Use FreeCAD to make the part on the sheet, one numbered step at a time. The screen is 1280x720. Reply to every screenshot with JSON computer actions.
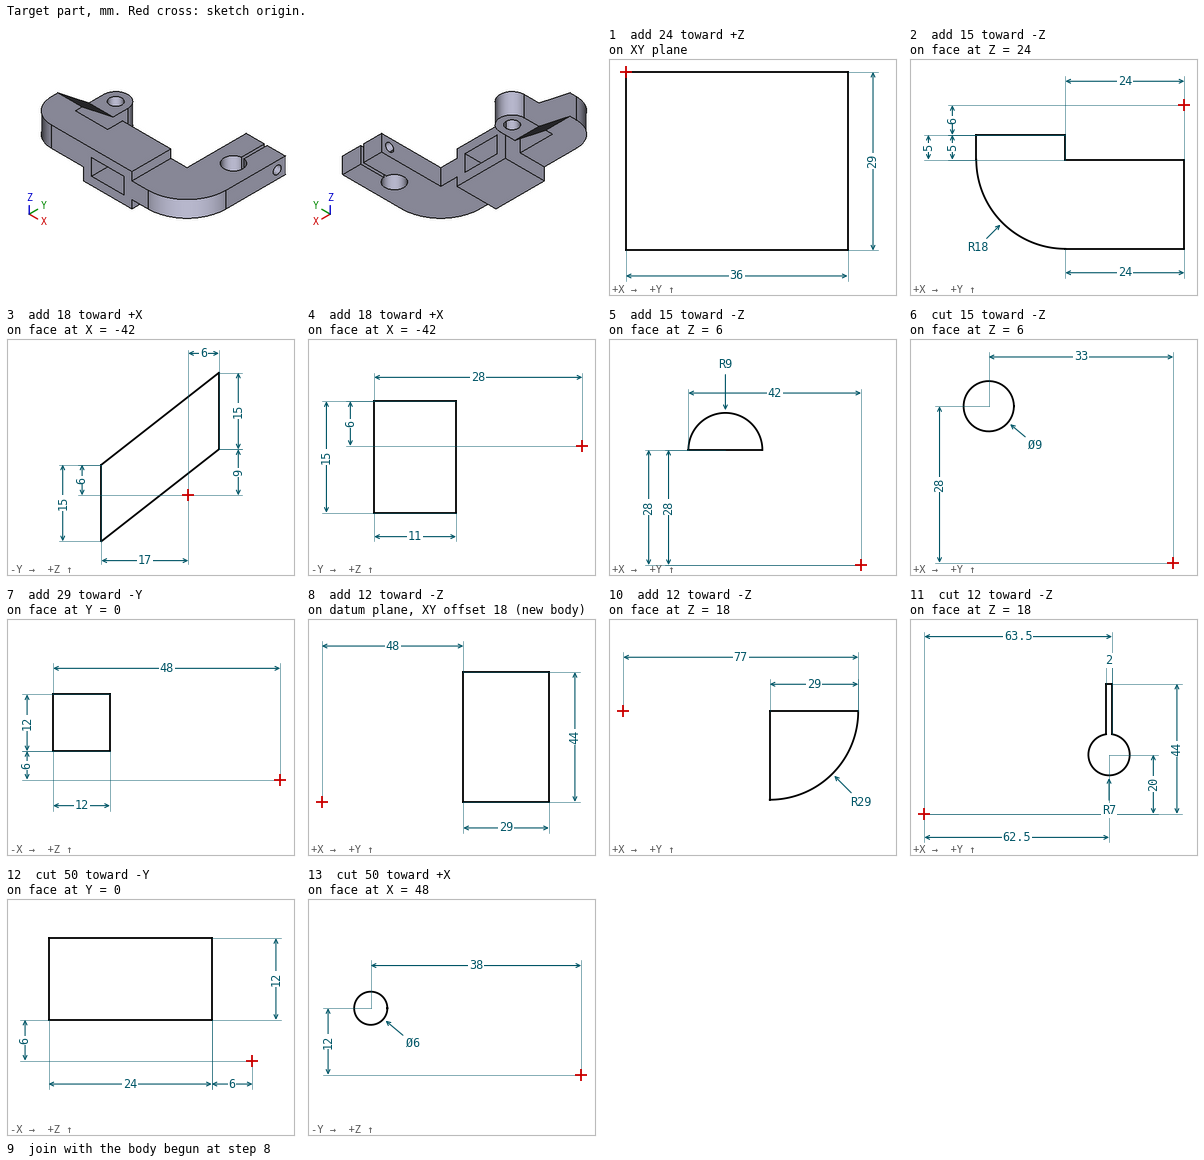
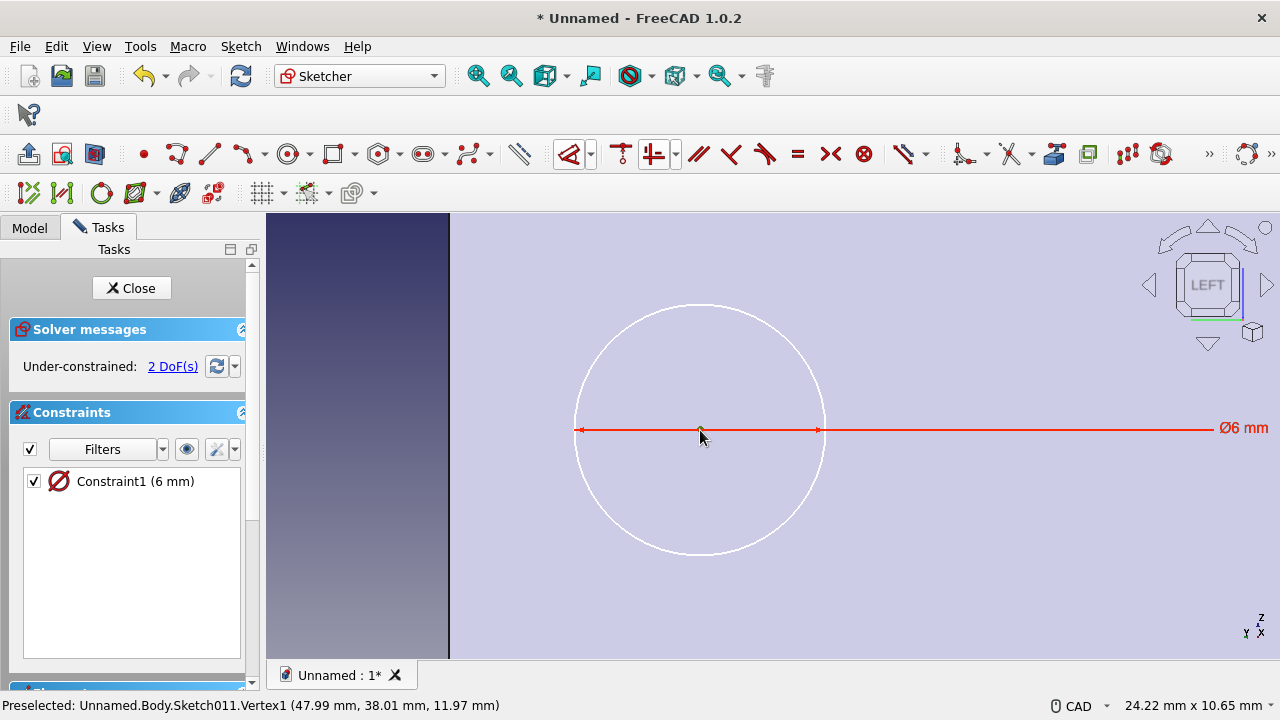
{"action": "key", "text": "l"}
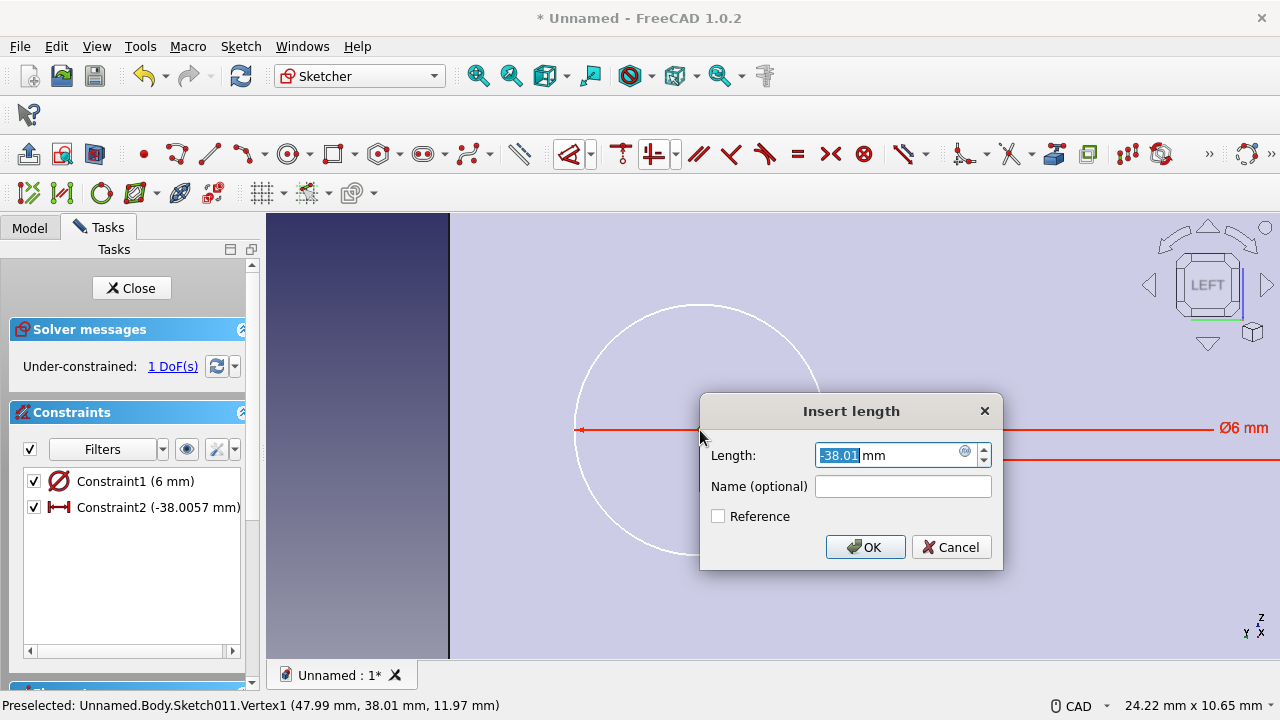
{"action": "type", "text": "-38"}
{"action": "key", "text": "Return"}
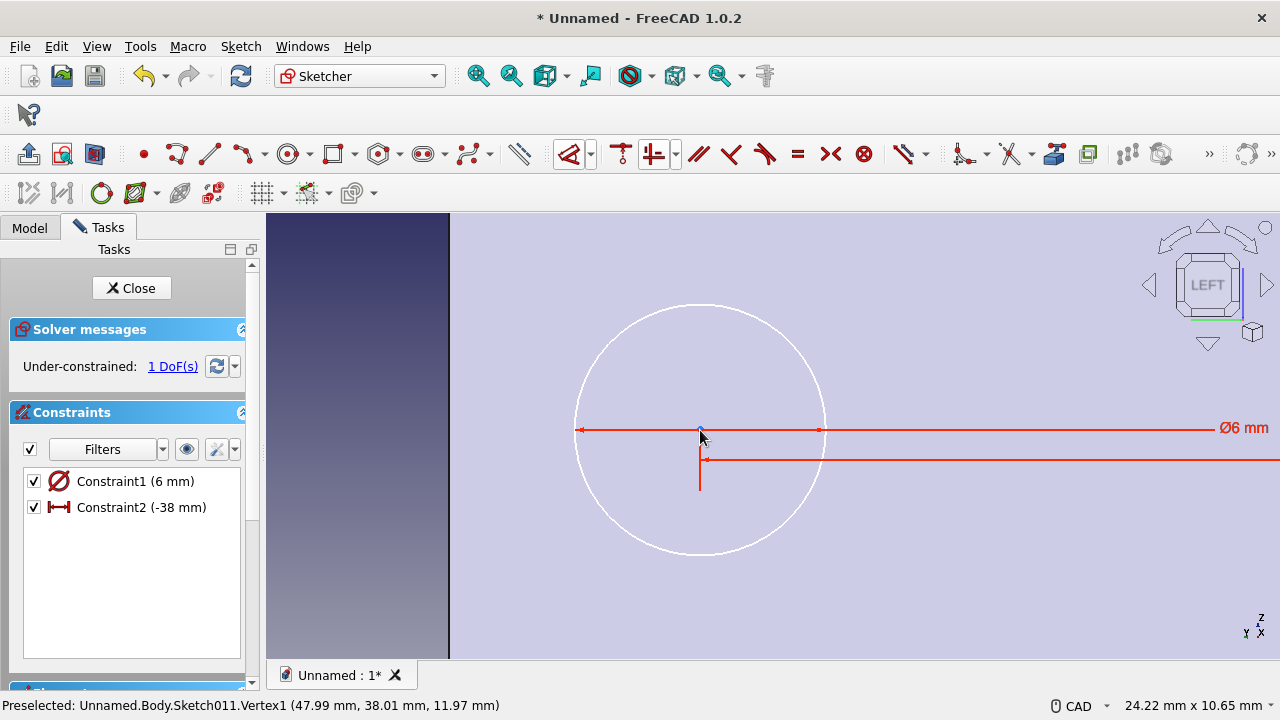
{"action": "left_click", "coordinate": [700, 430]}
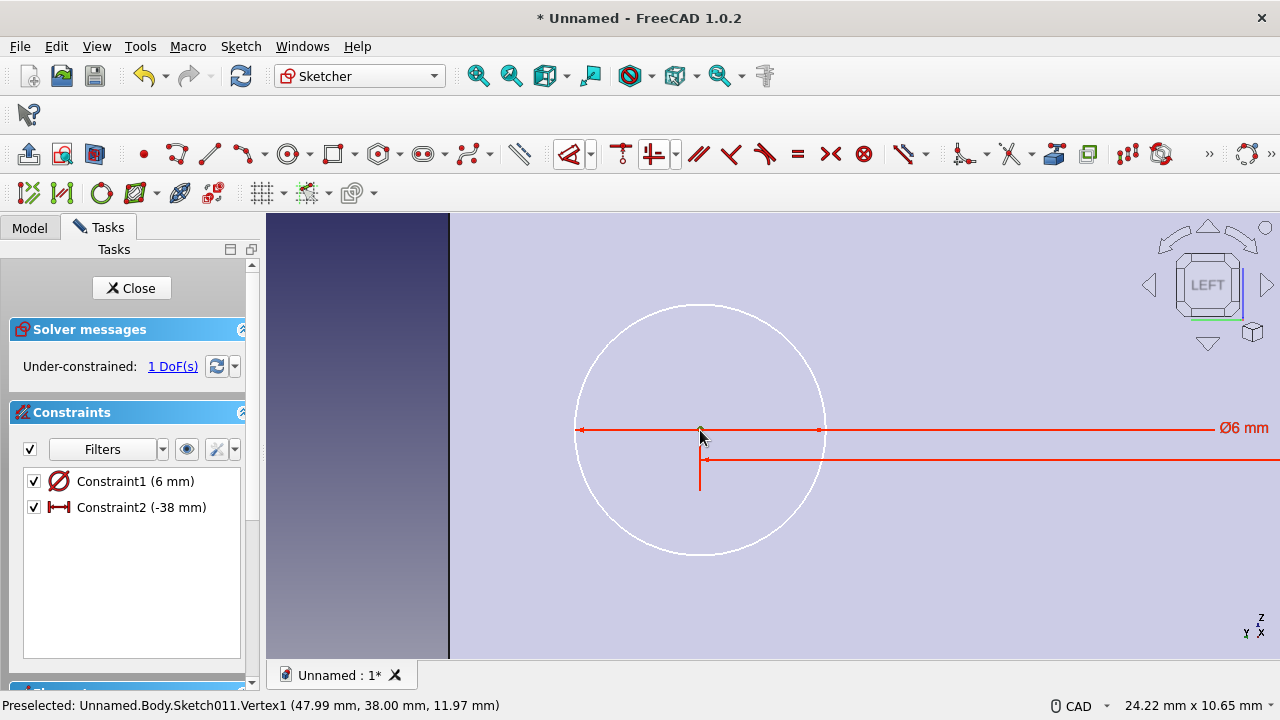
{"action": "left_click", "coordinate": [590, 154]}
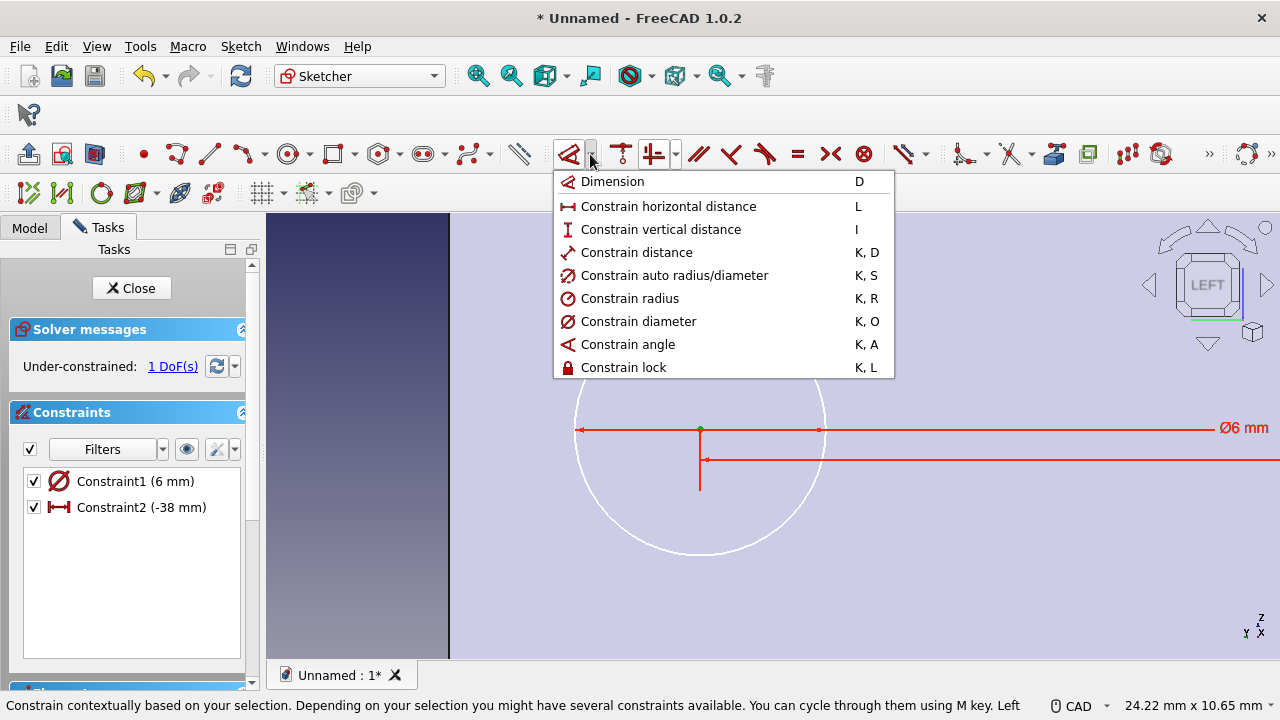
{"action": "left_click", "coordinate": [724, 230]}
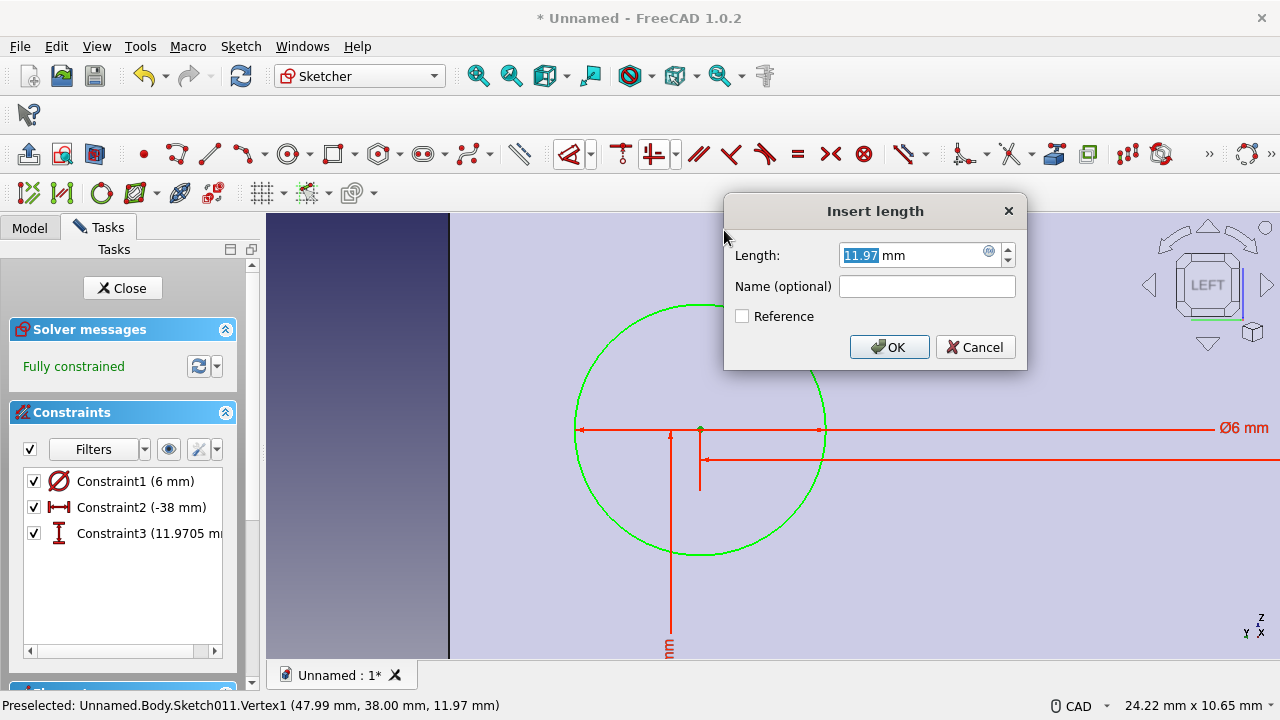
{"action": "type", "text": "12"}
{"action": "key", "text": "Return"}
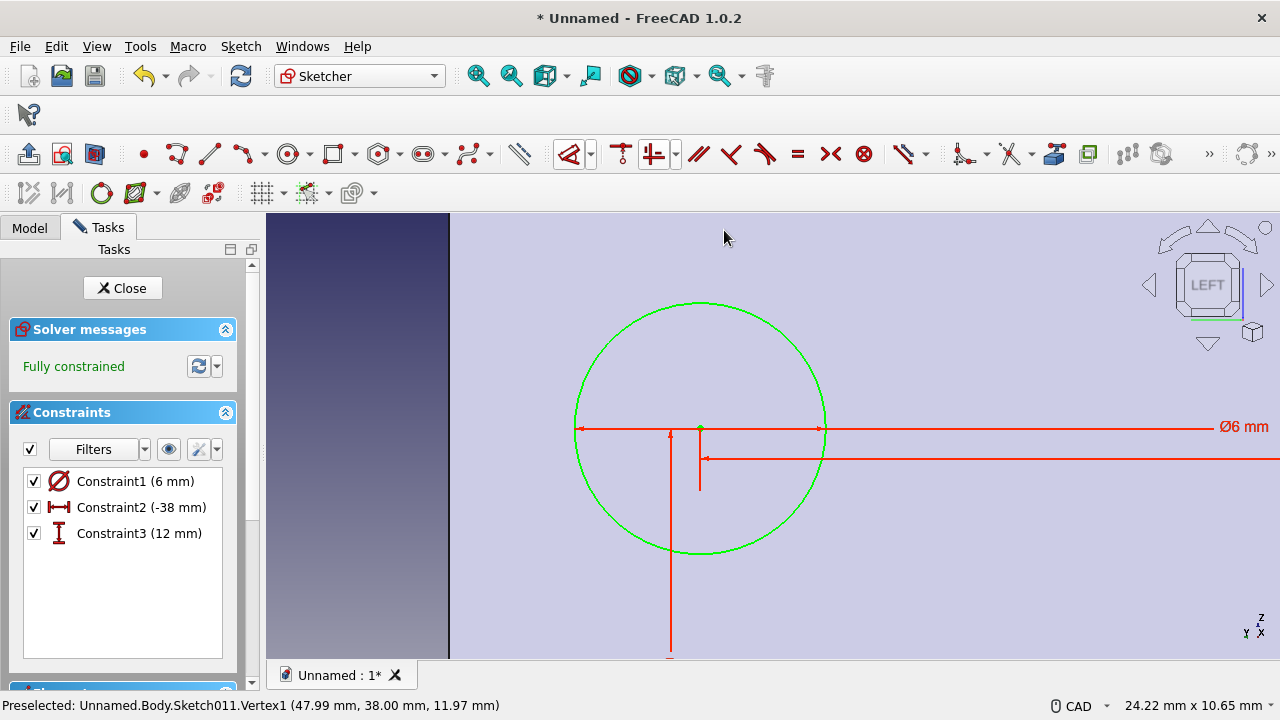
{"action": "left_click", "coordinate": [123, 288]}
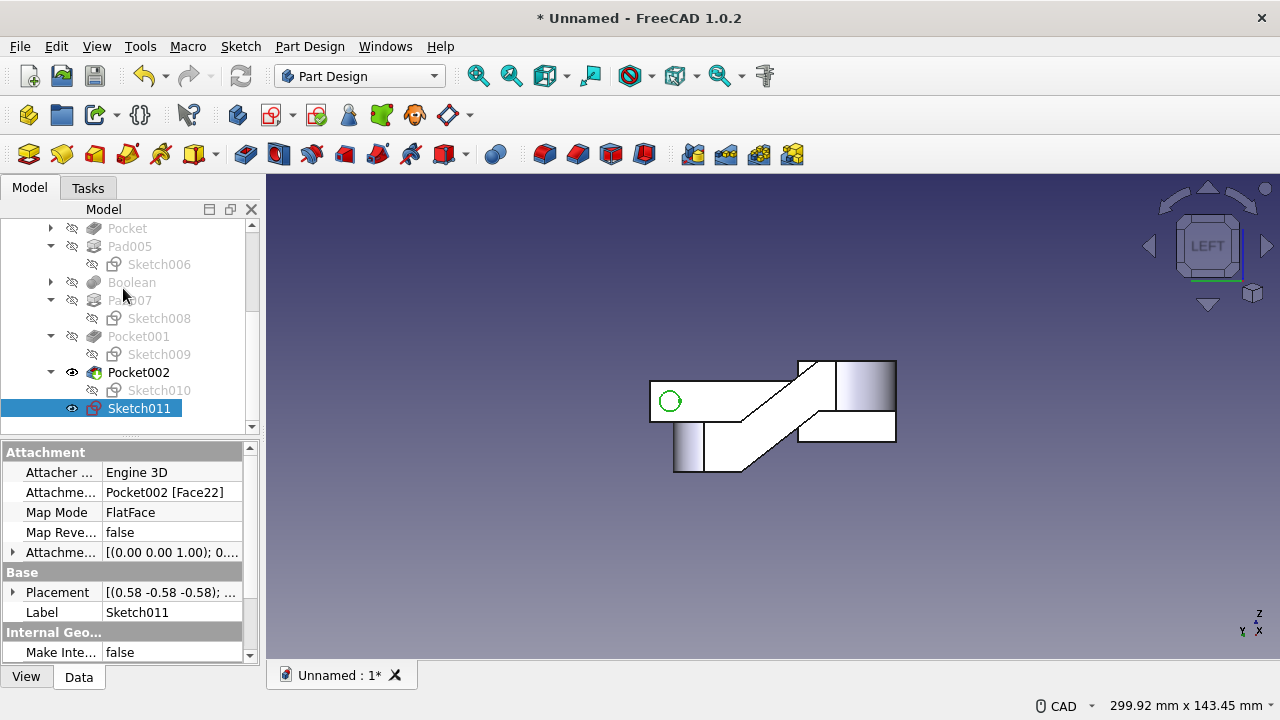
{"action": "left_click", "coordinate": [246, 154]}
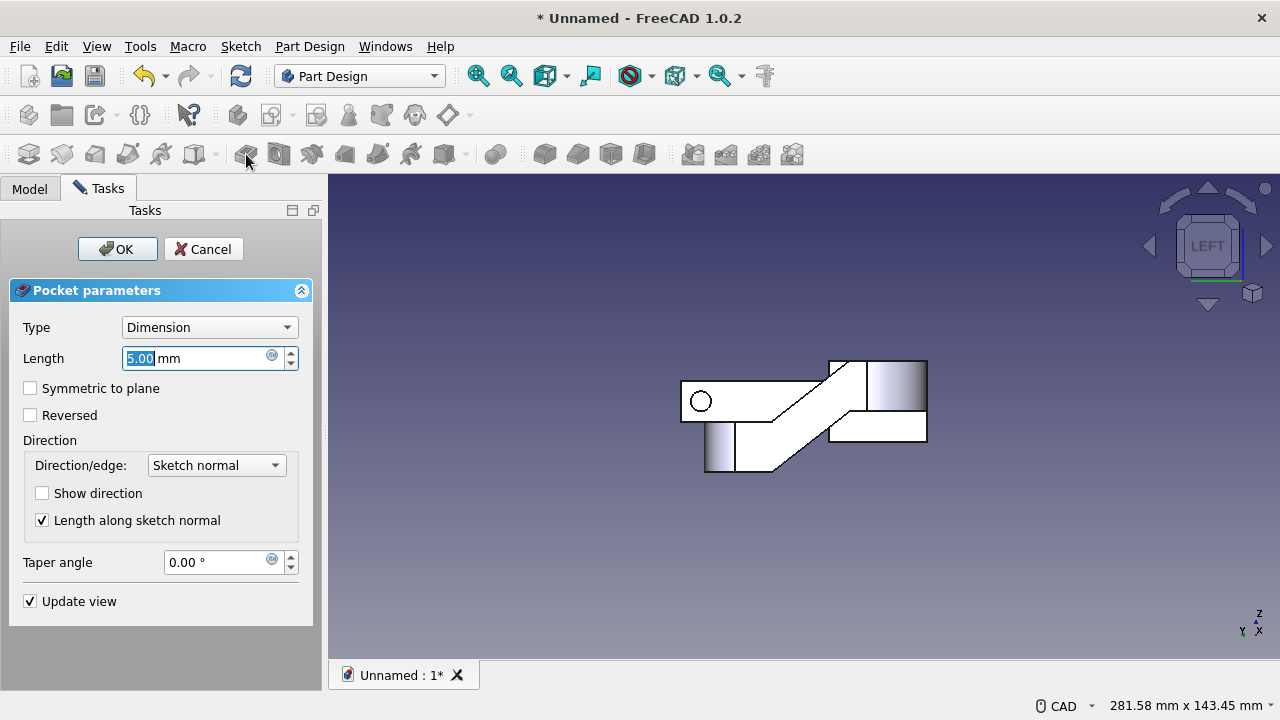
{"action": "type", "text": "50"}
{"action": "key", "text": "Tab"}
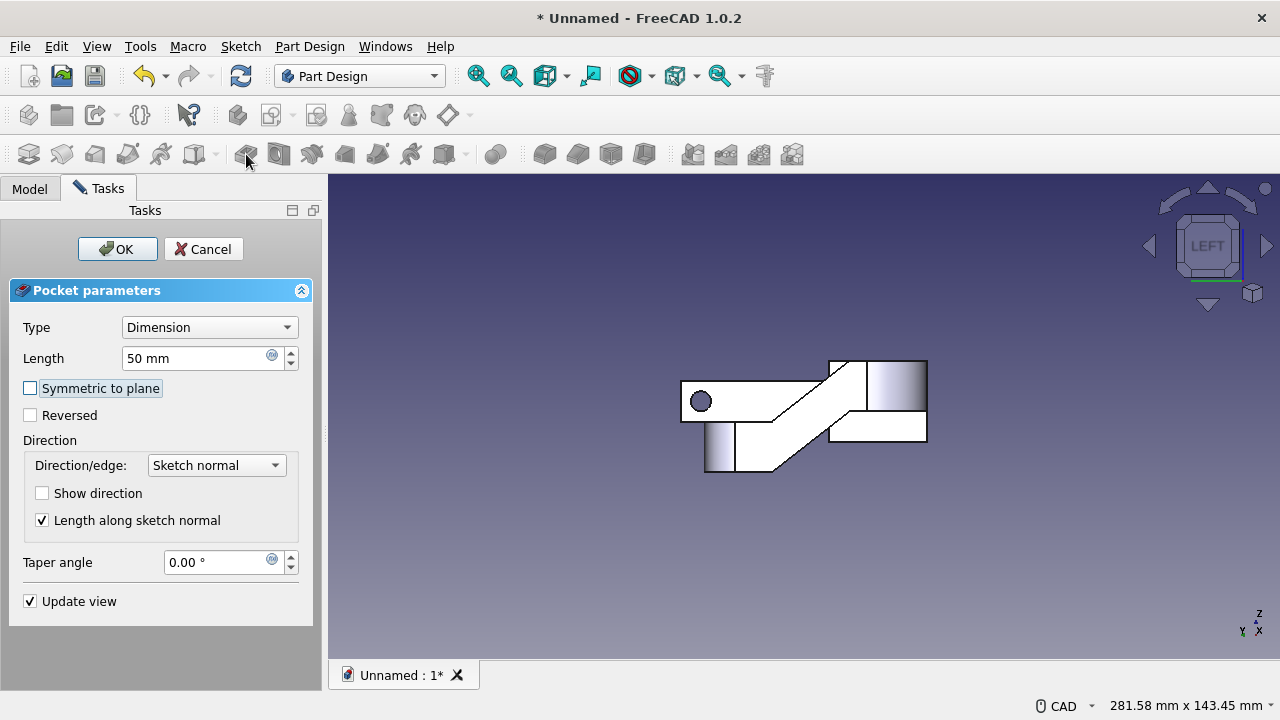
{"action": "left_click", "coordinate": [118, 249]}